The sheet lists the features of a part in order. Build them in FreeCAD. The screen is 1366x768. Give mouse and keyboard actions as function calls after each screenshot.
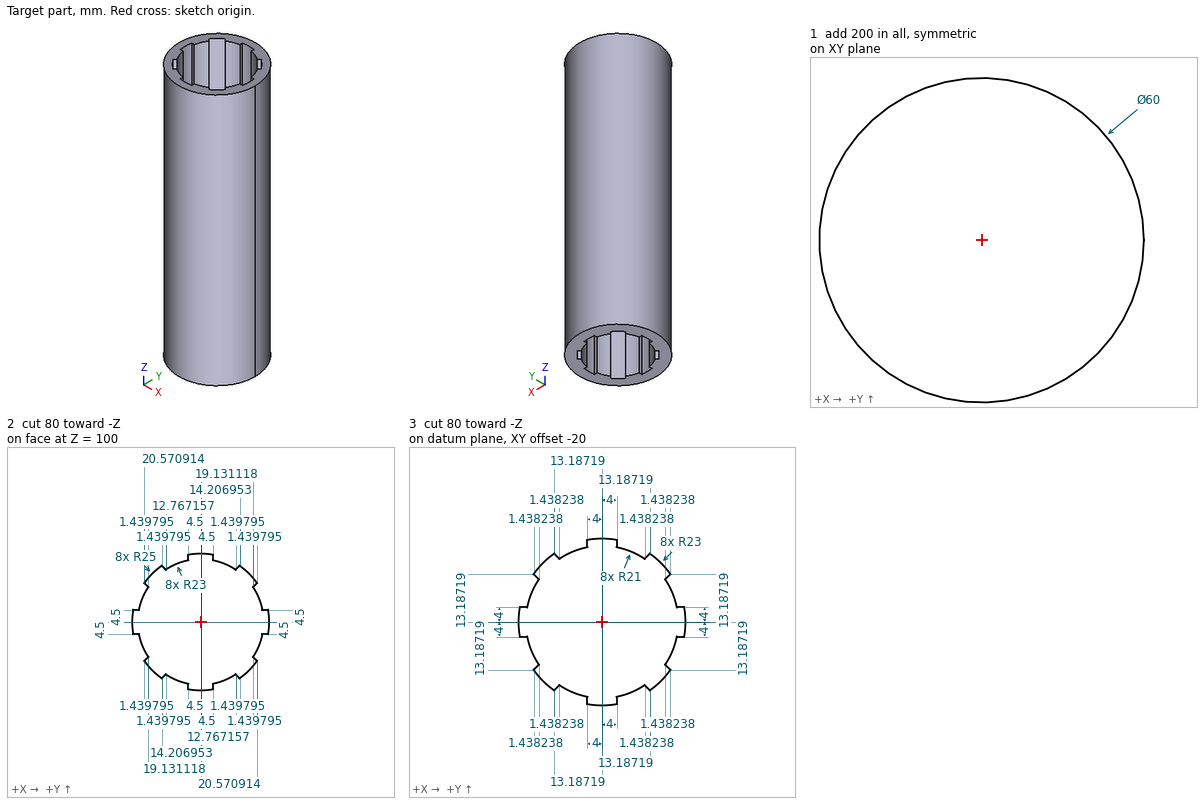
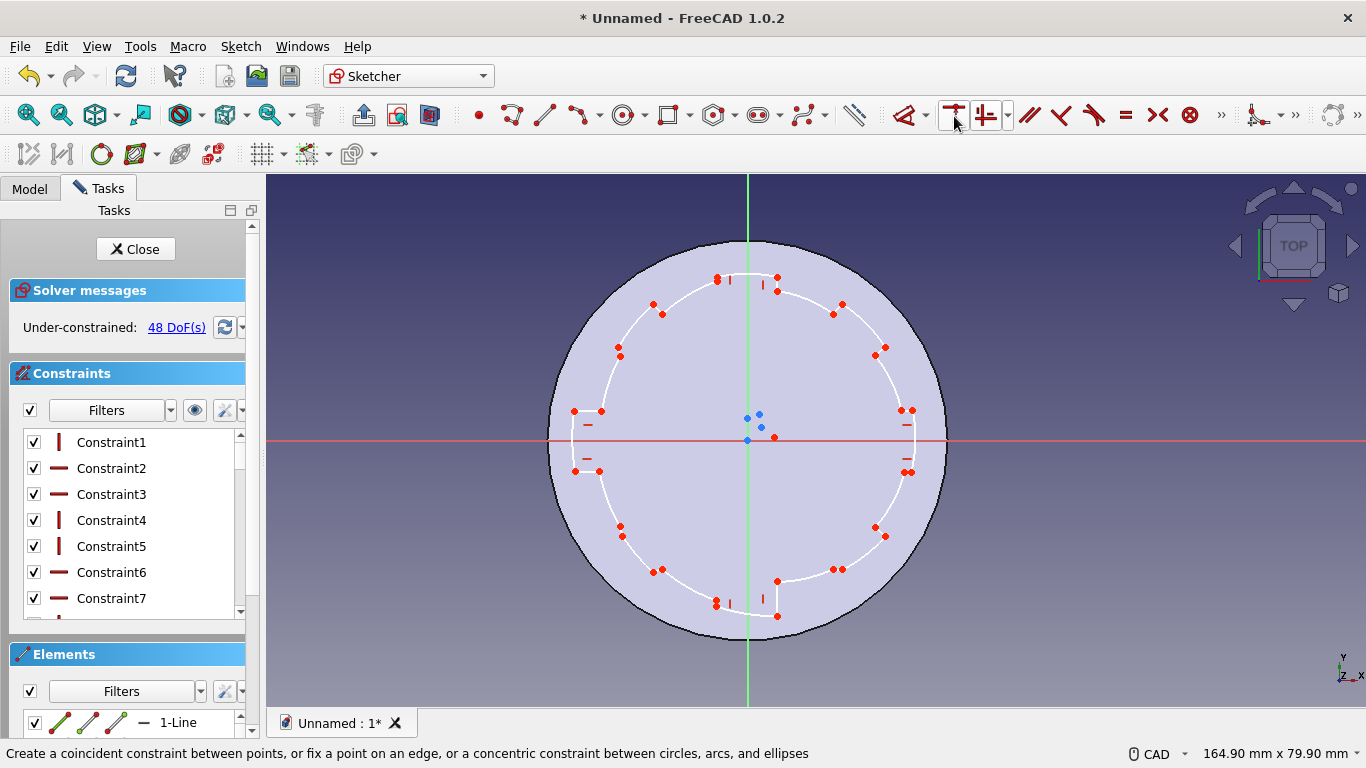
click(699, 289)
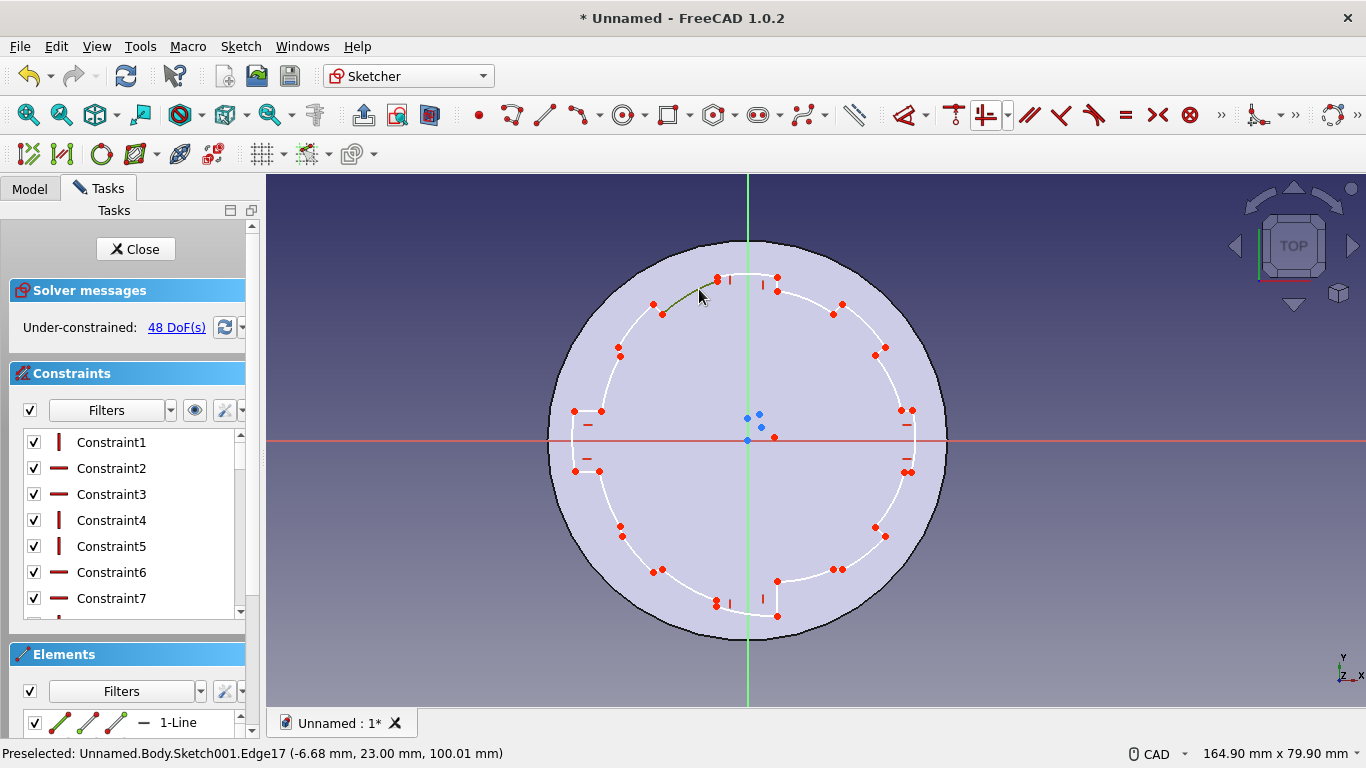
click(874, 332)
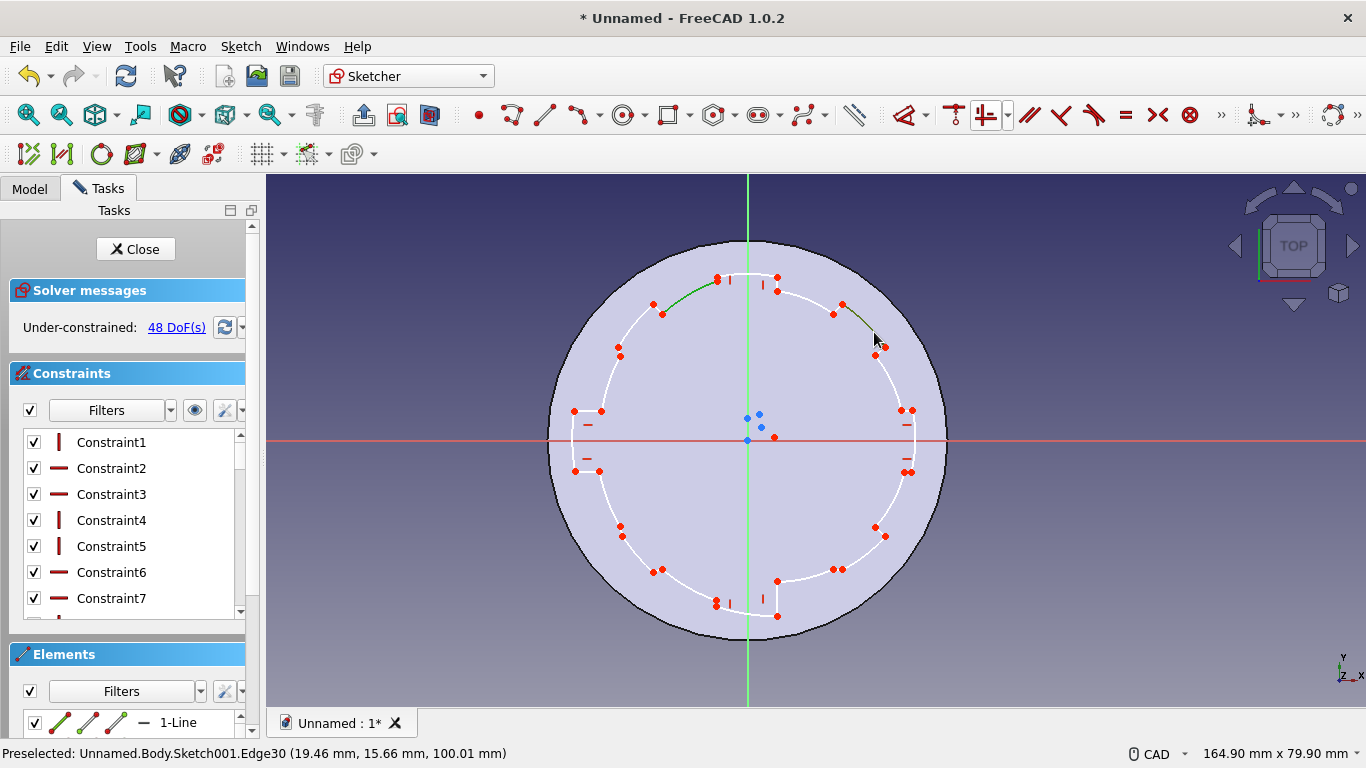
click(954, 116)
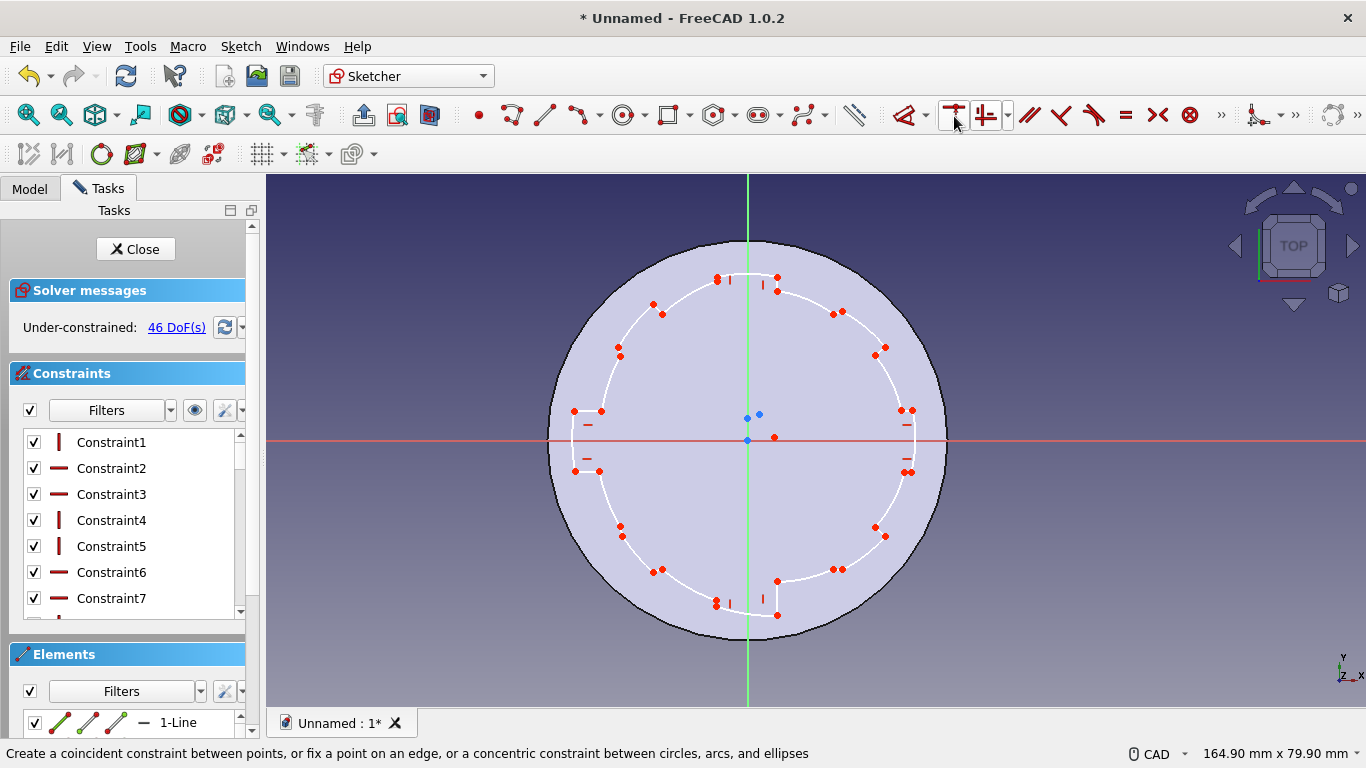
click(699, 289)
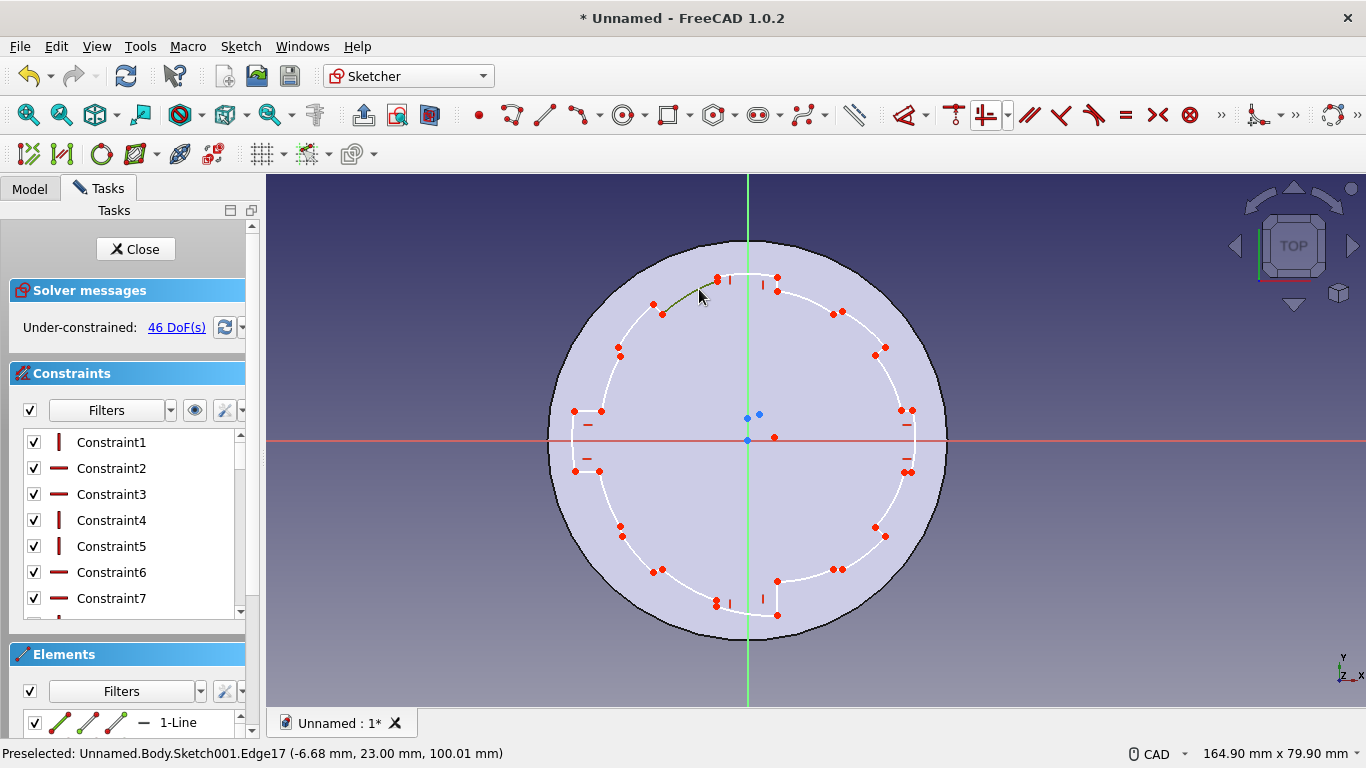
click(818, 304)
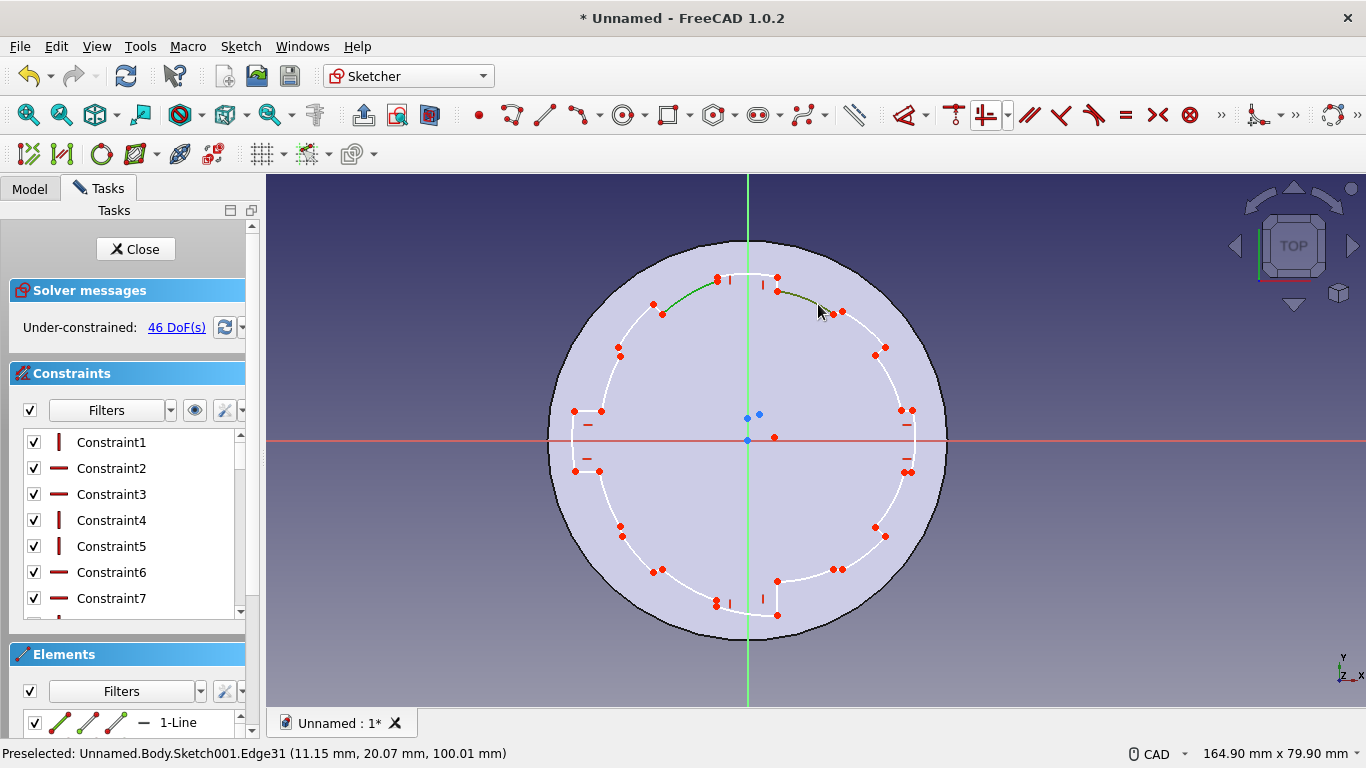
click(954, 116)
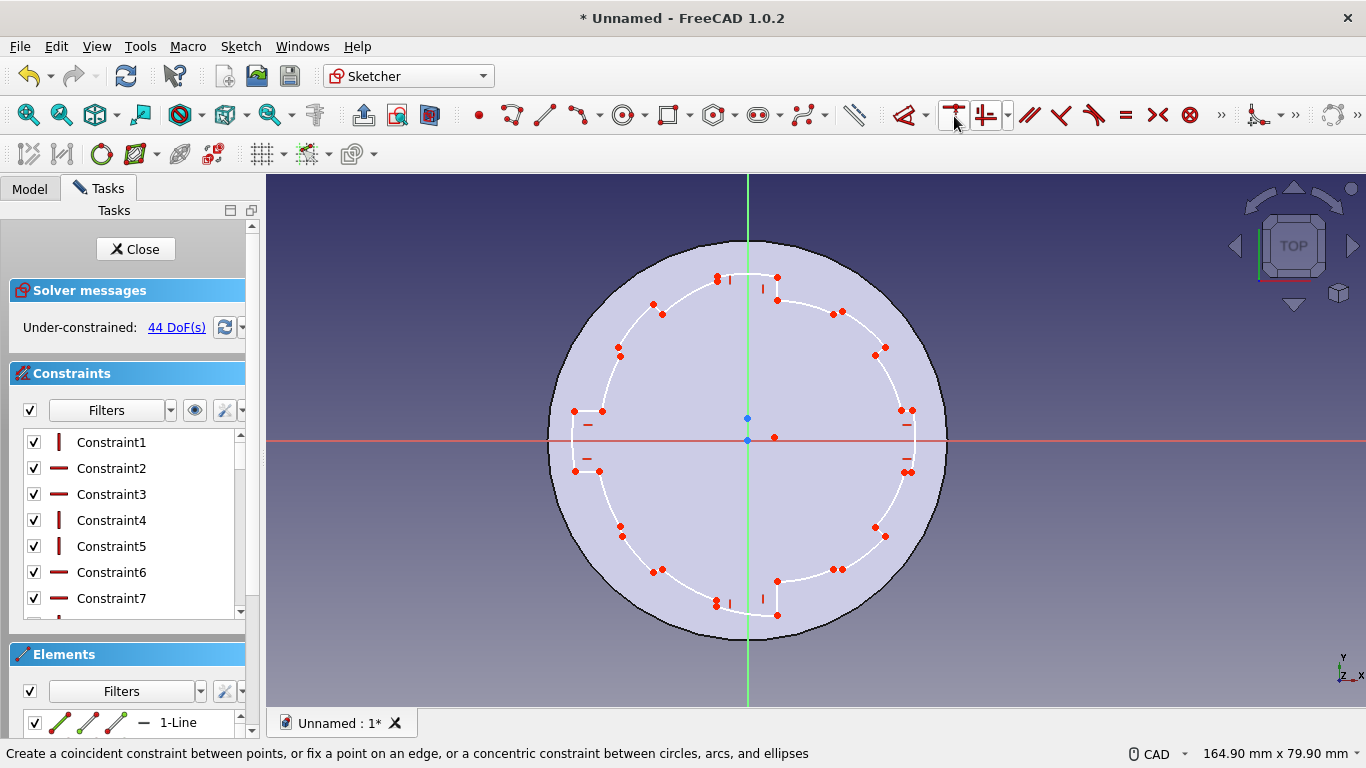
click(699, 289)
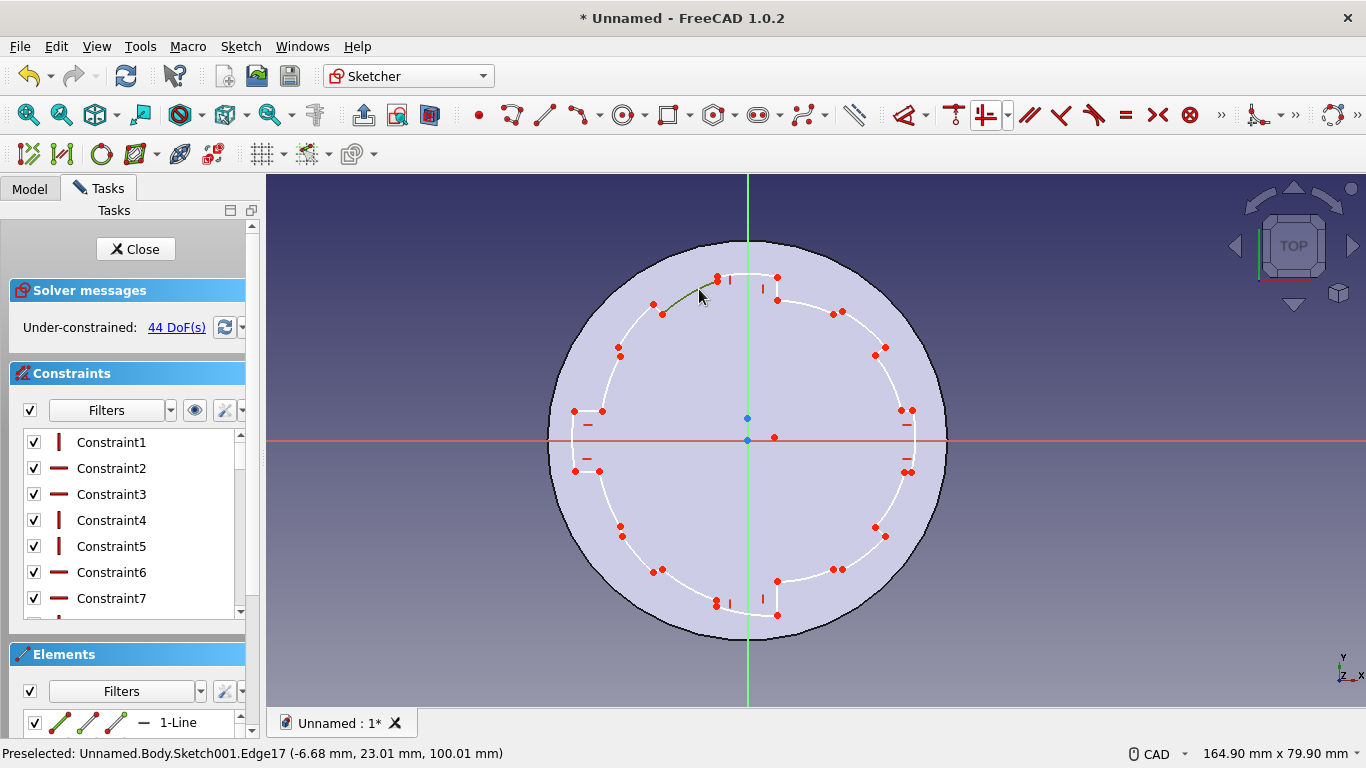
click(759, 274)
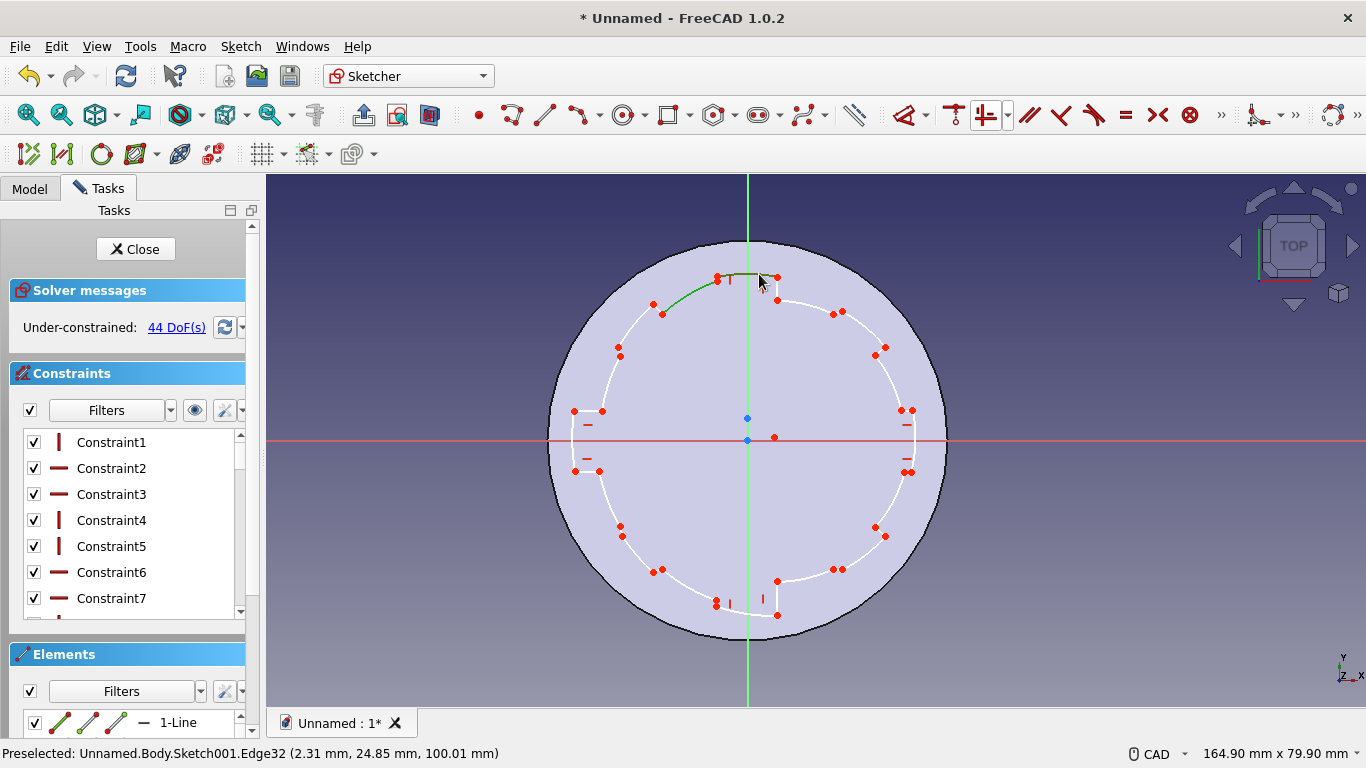
click(954, 116)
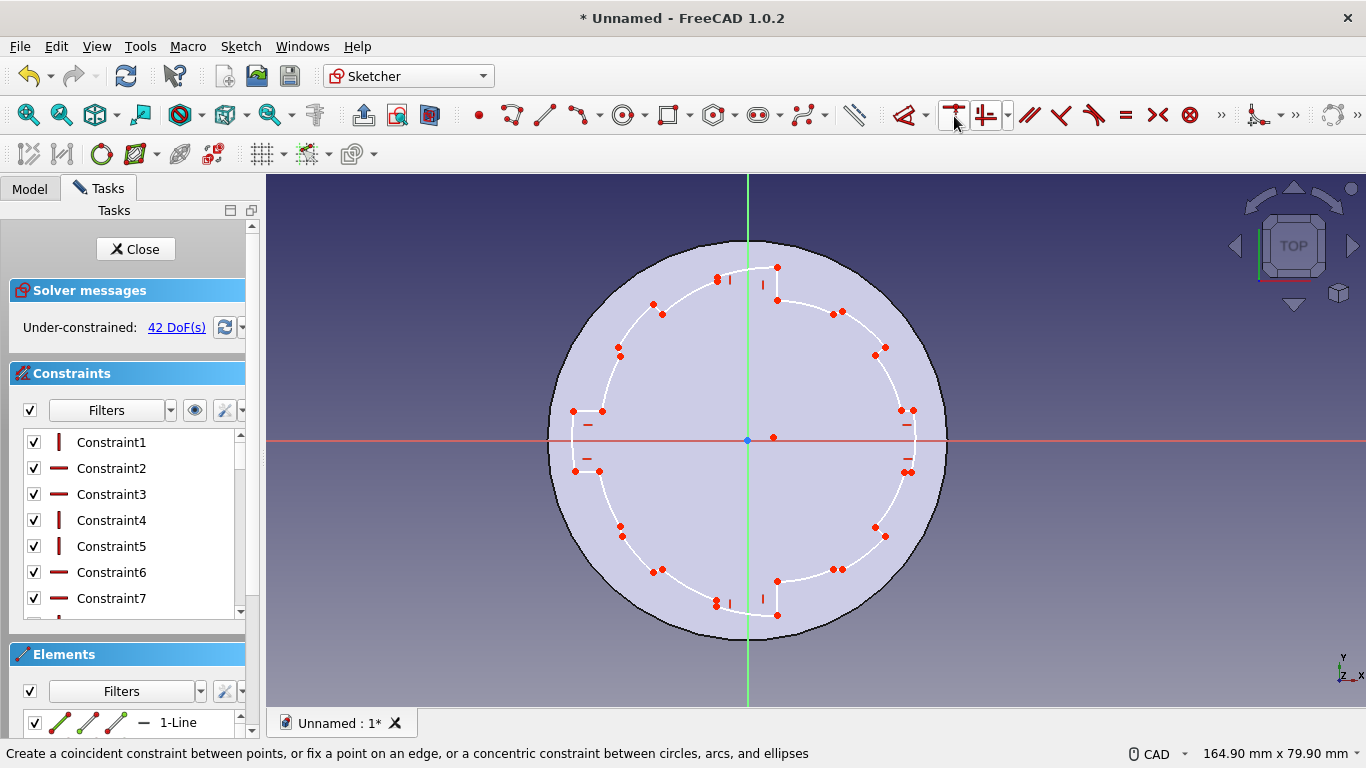
drag(738, 428, 784, 451)